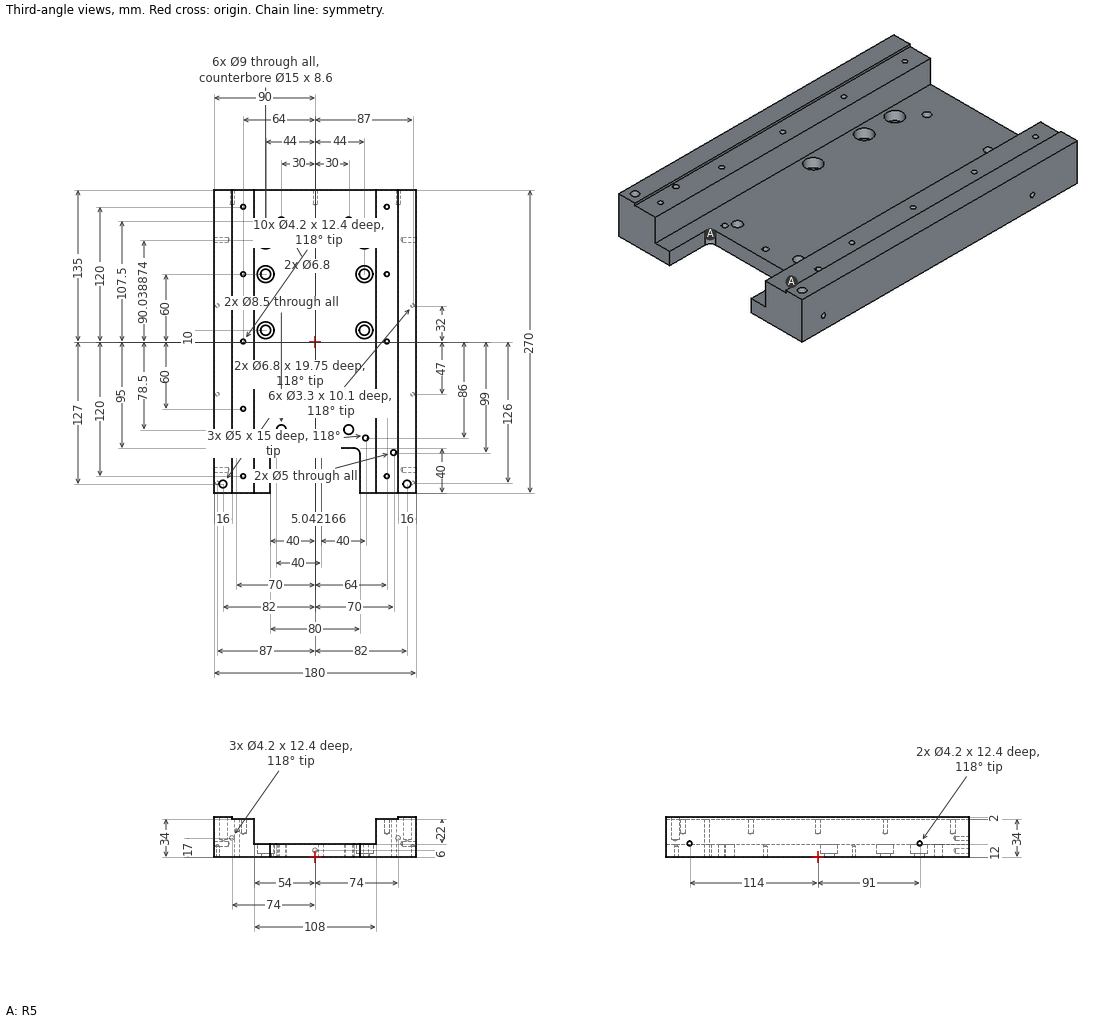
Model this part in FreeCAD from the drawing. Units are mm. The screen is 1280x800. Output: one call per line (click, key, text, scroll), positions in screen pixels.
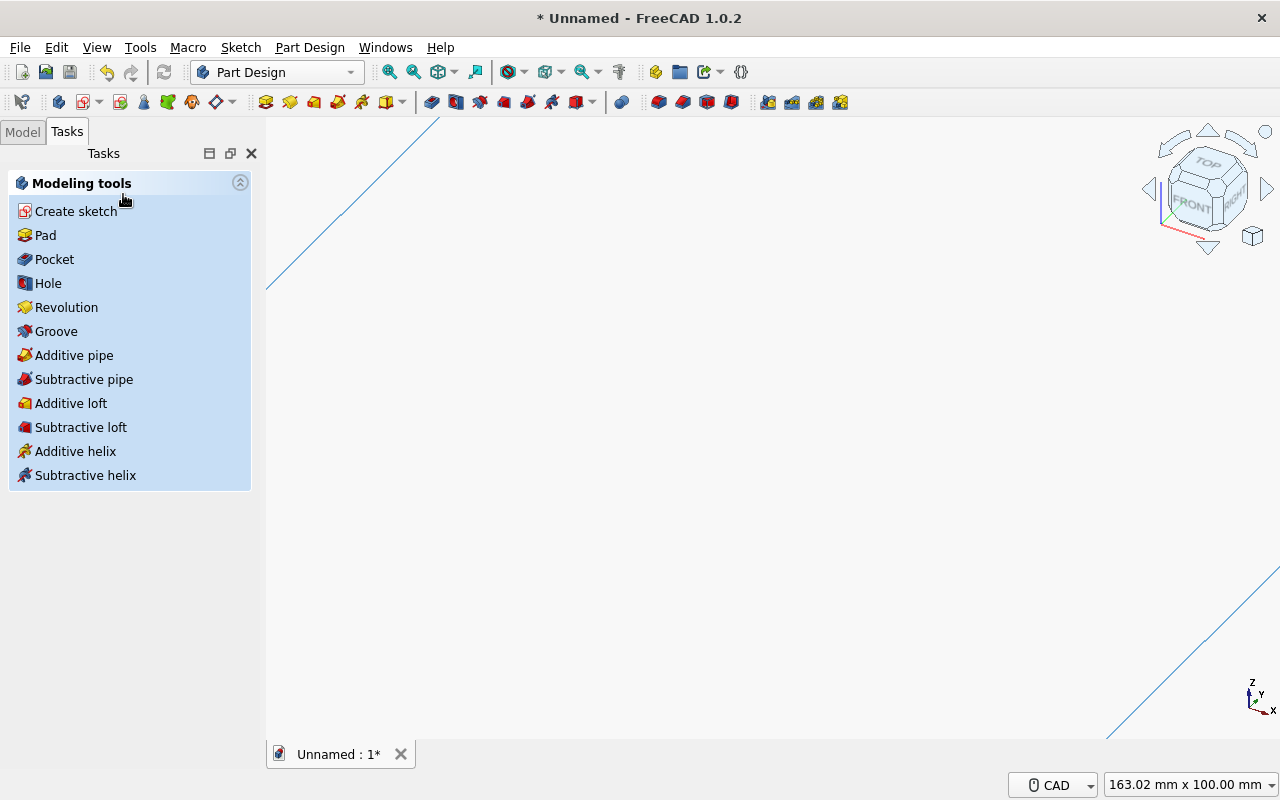
click(266, 102)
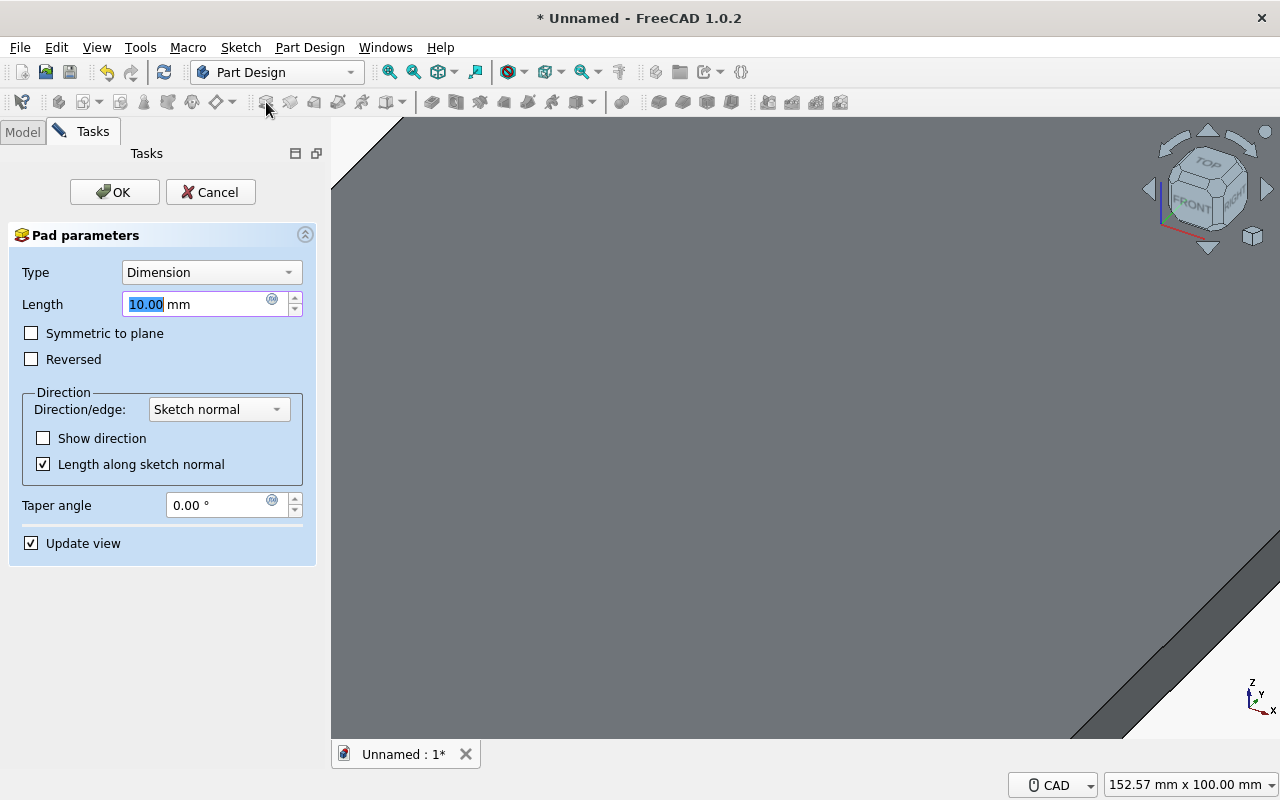
text(34)
key(Tab)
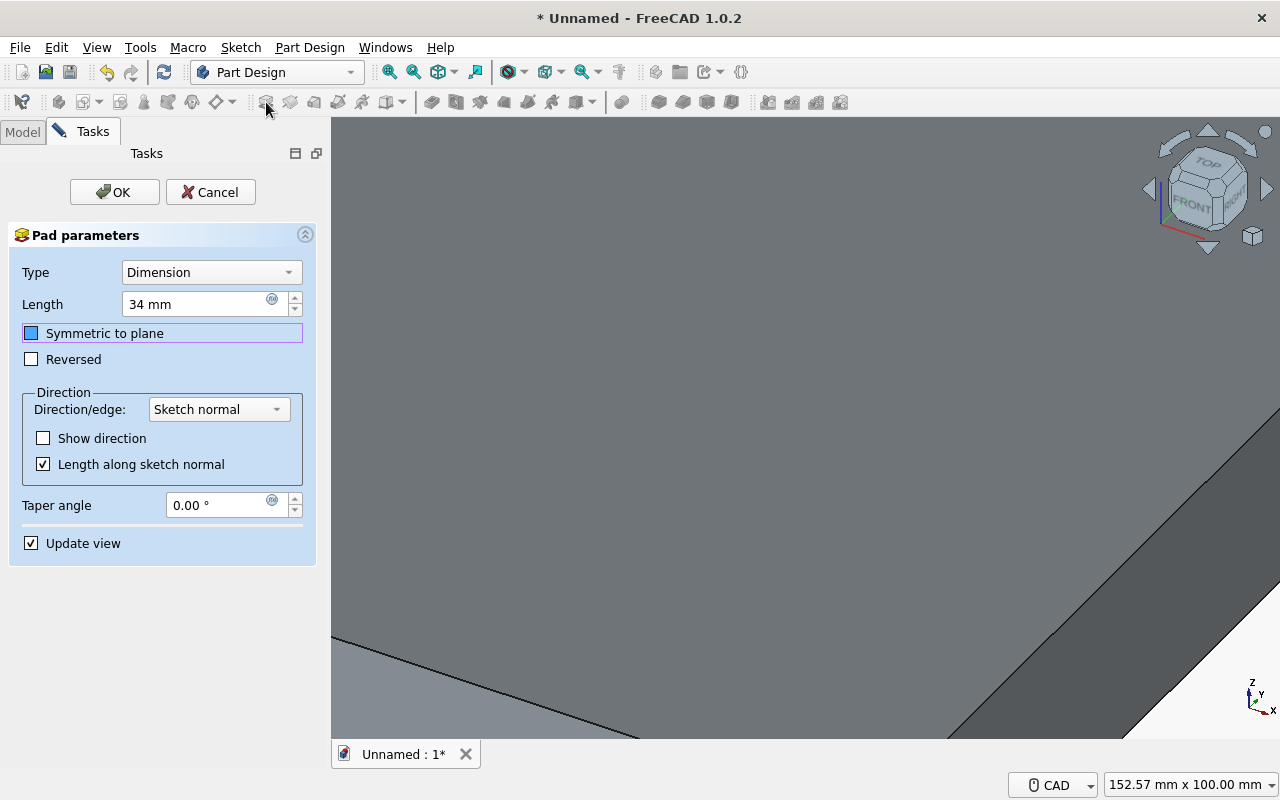
click(115, 192)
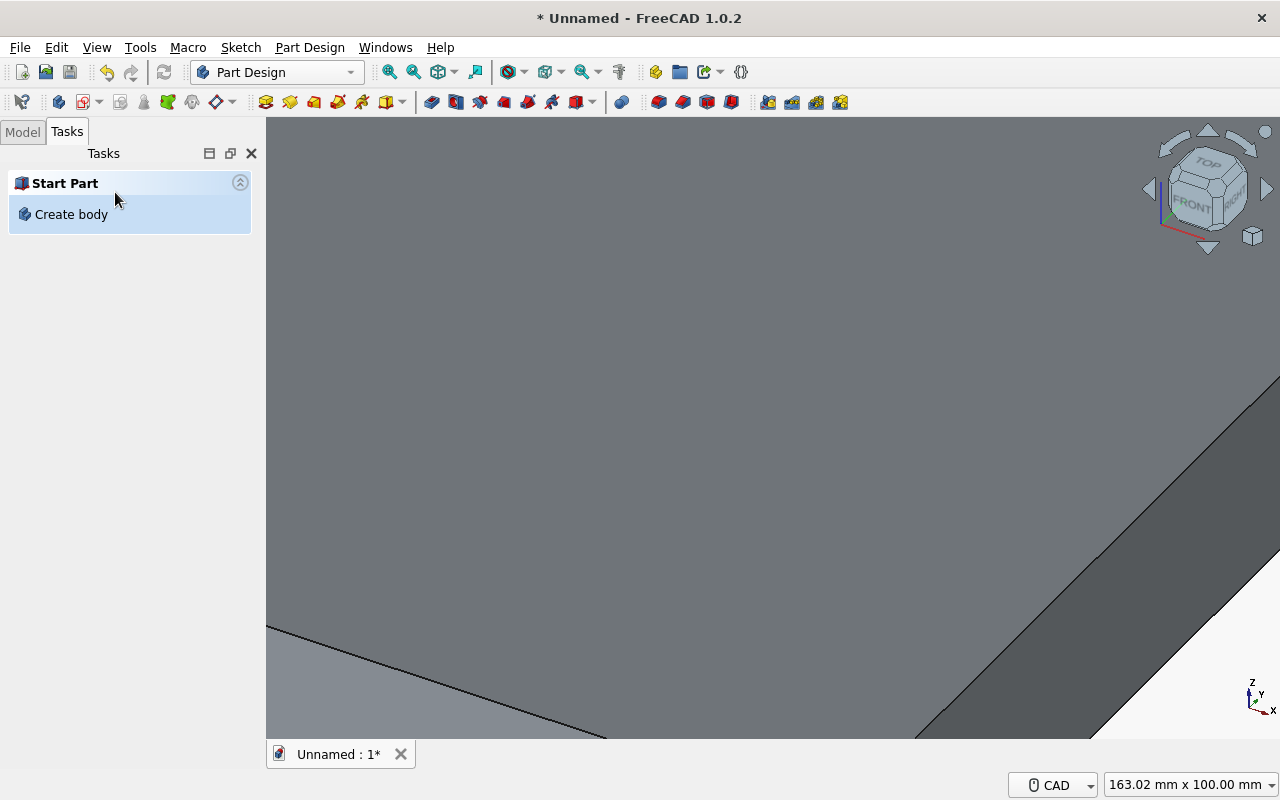
click(390, 72)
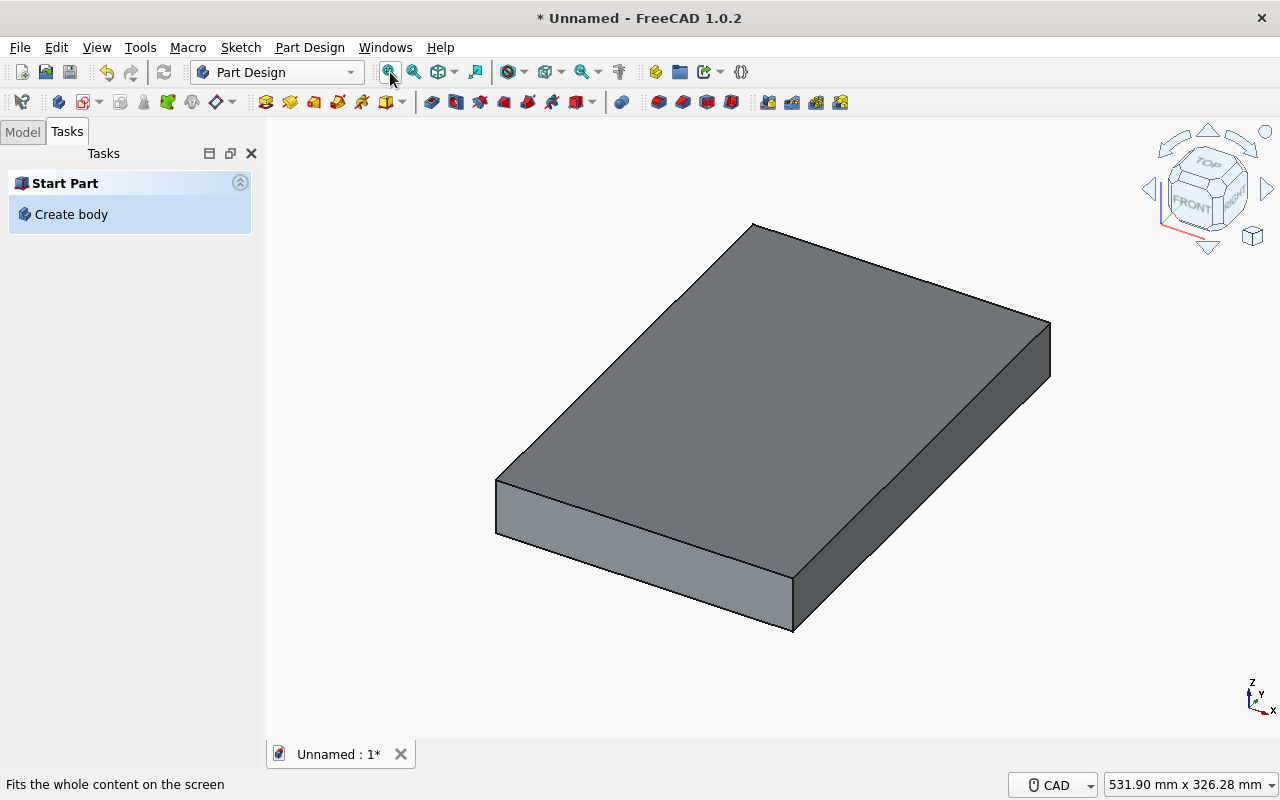
click(729, 583)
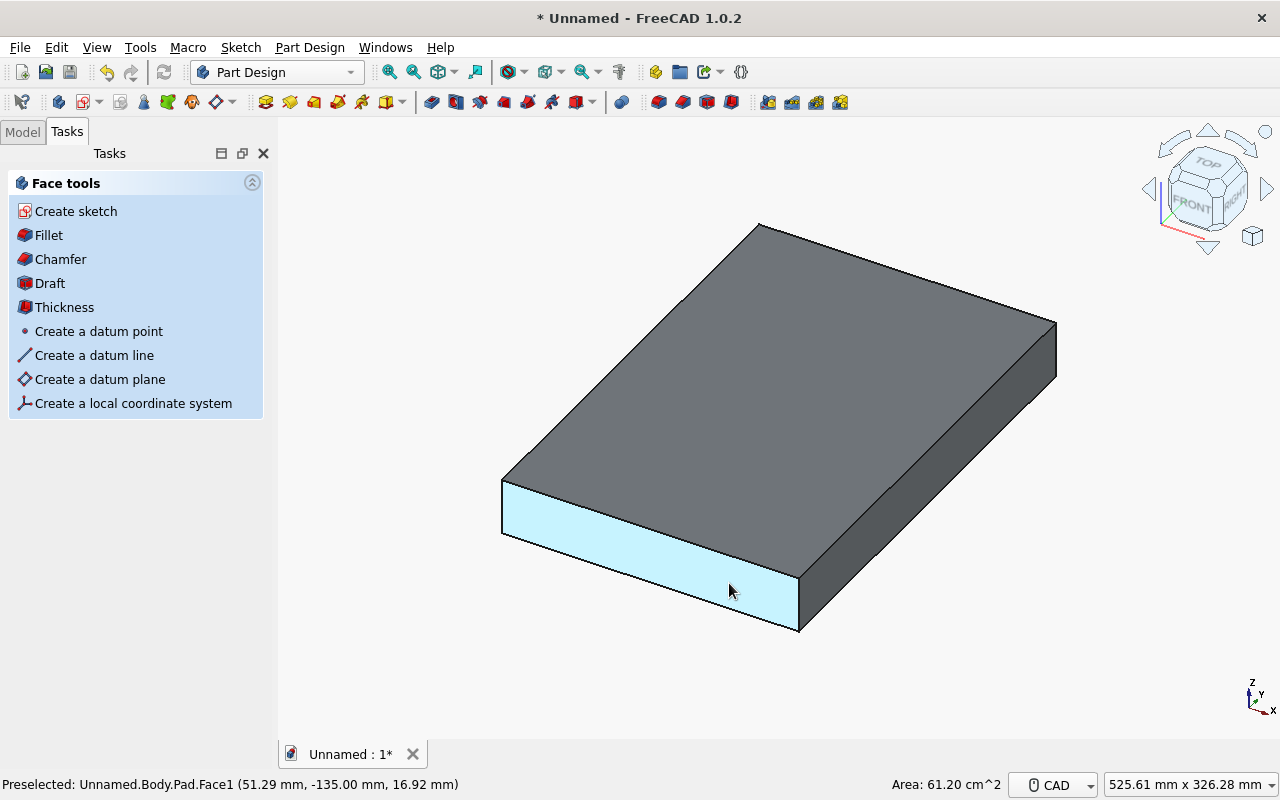
click(84, 102)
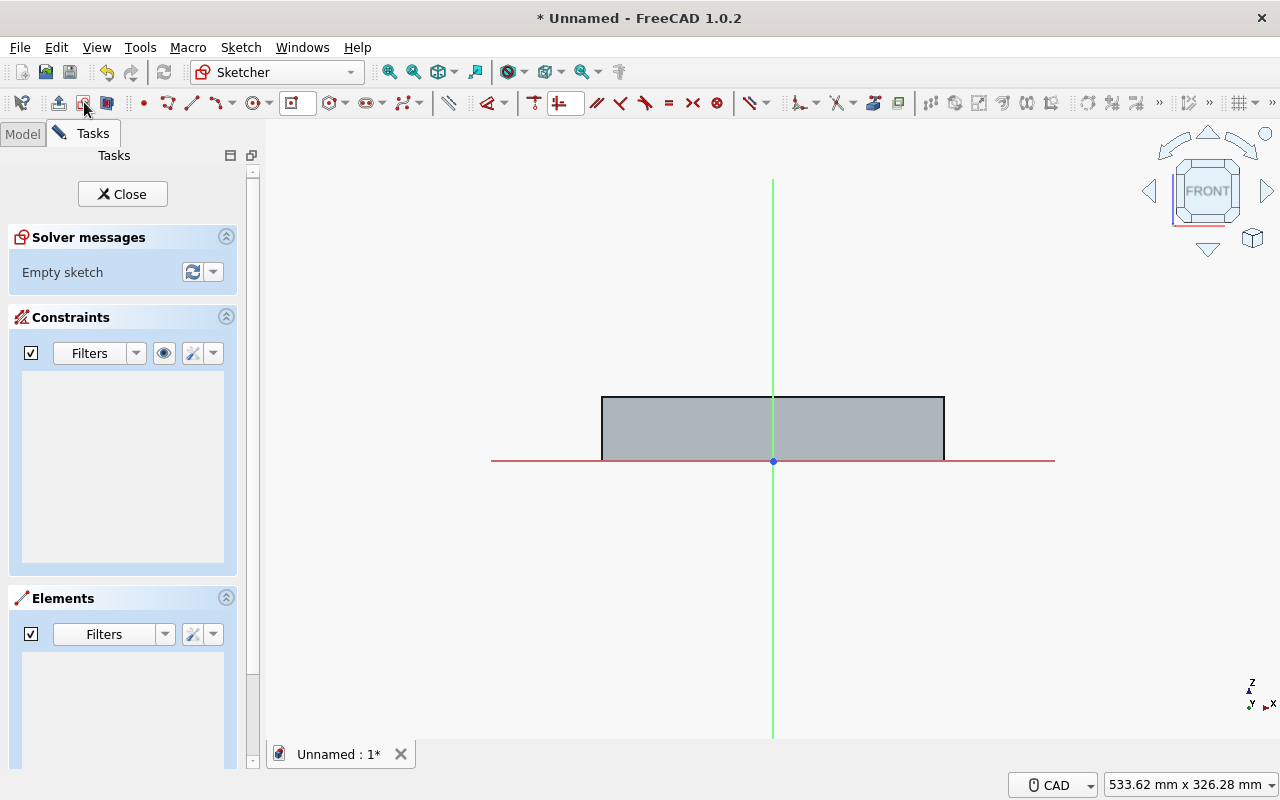
scroll(813, 429, up, 5)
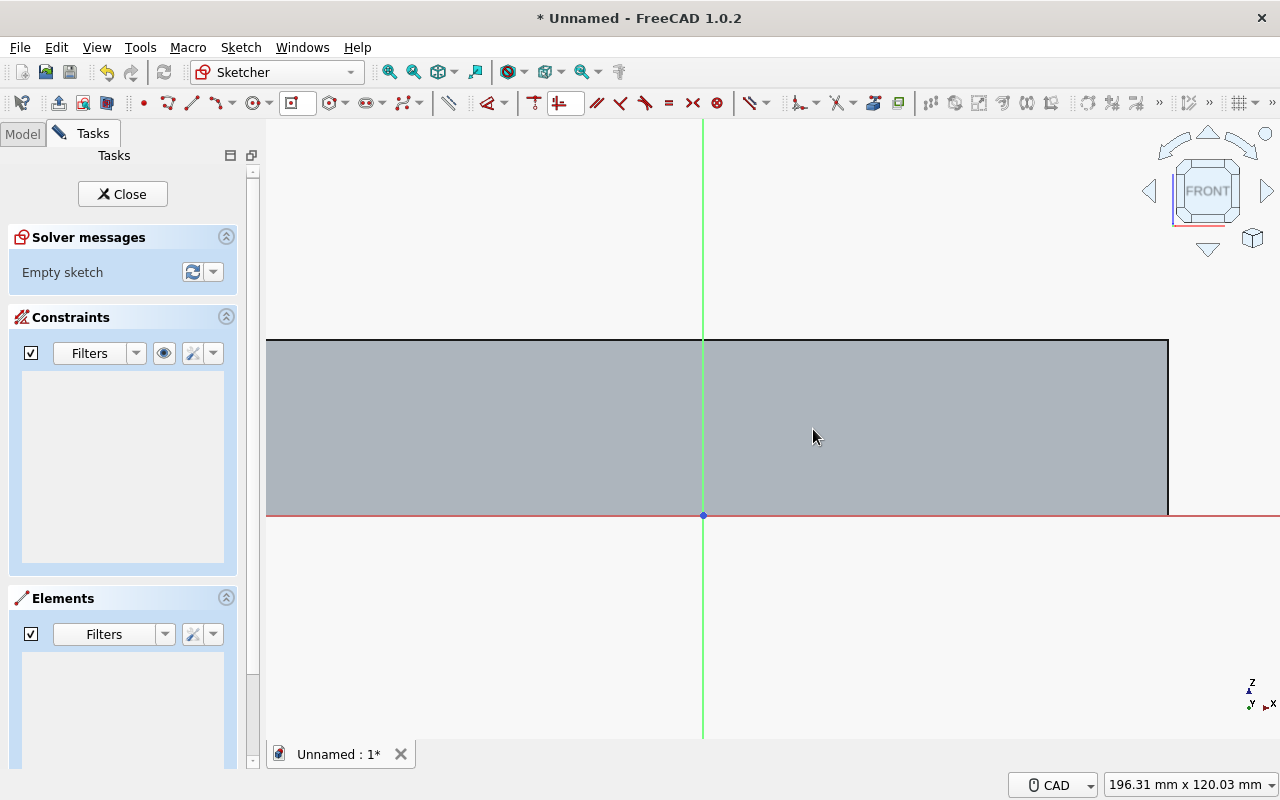
click(310, 104)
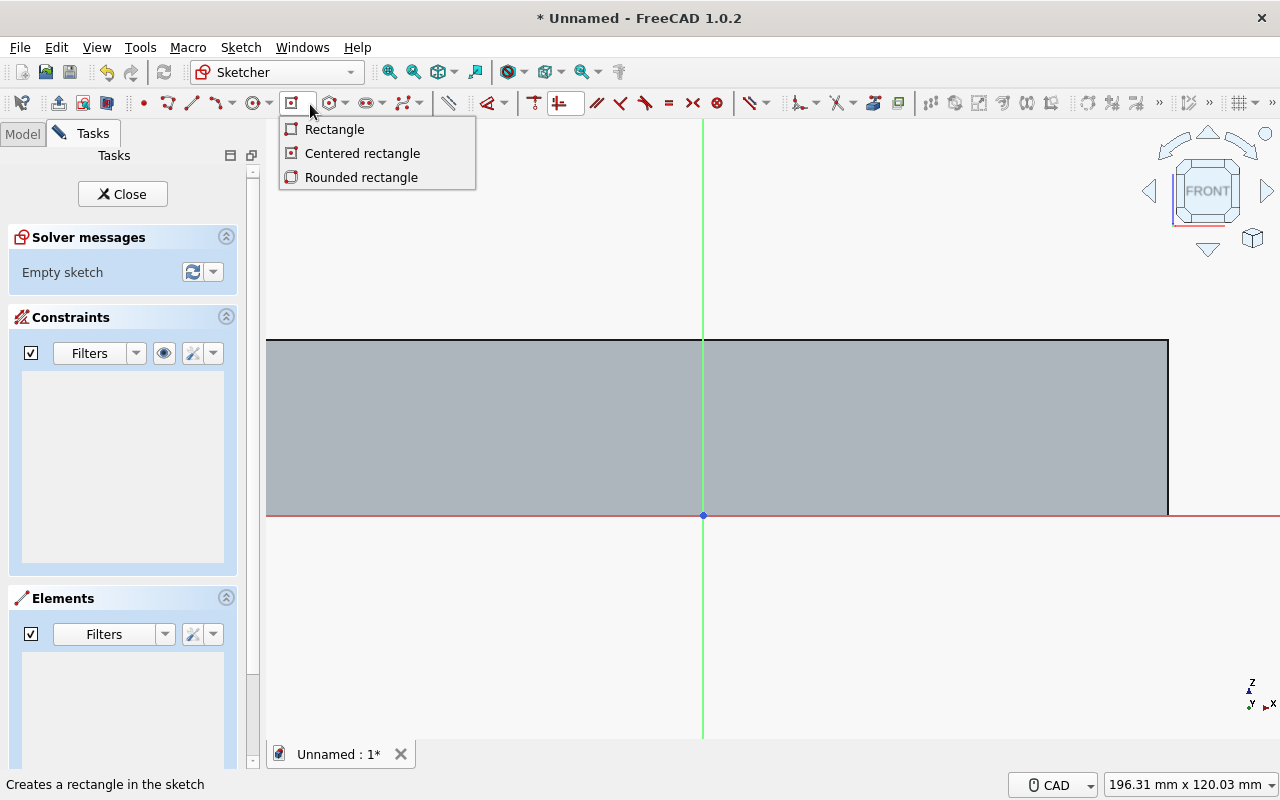
click(378, 129)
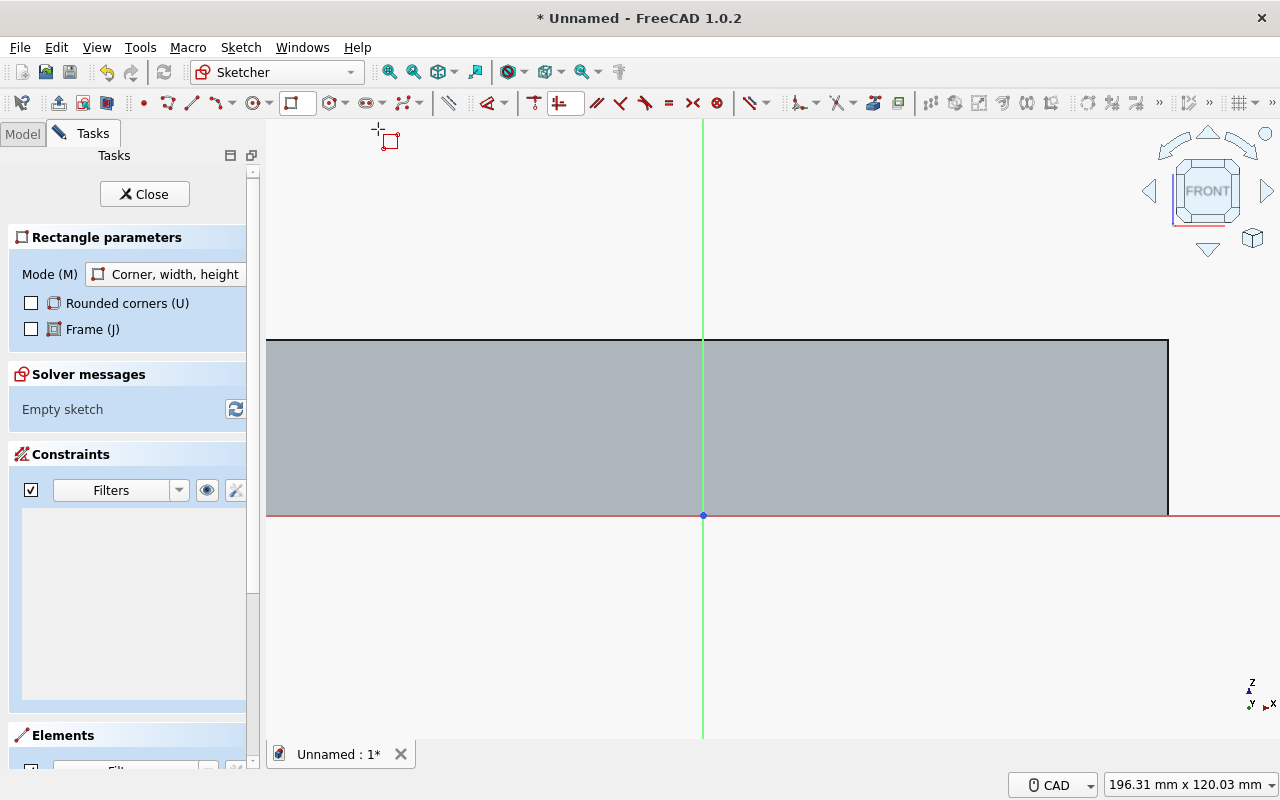
click(424, 340)
move(982, 454)